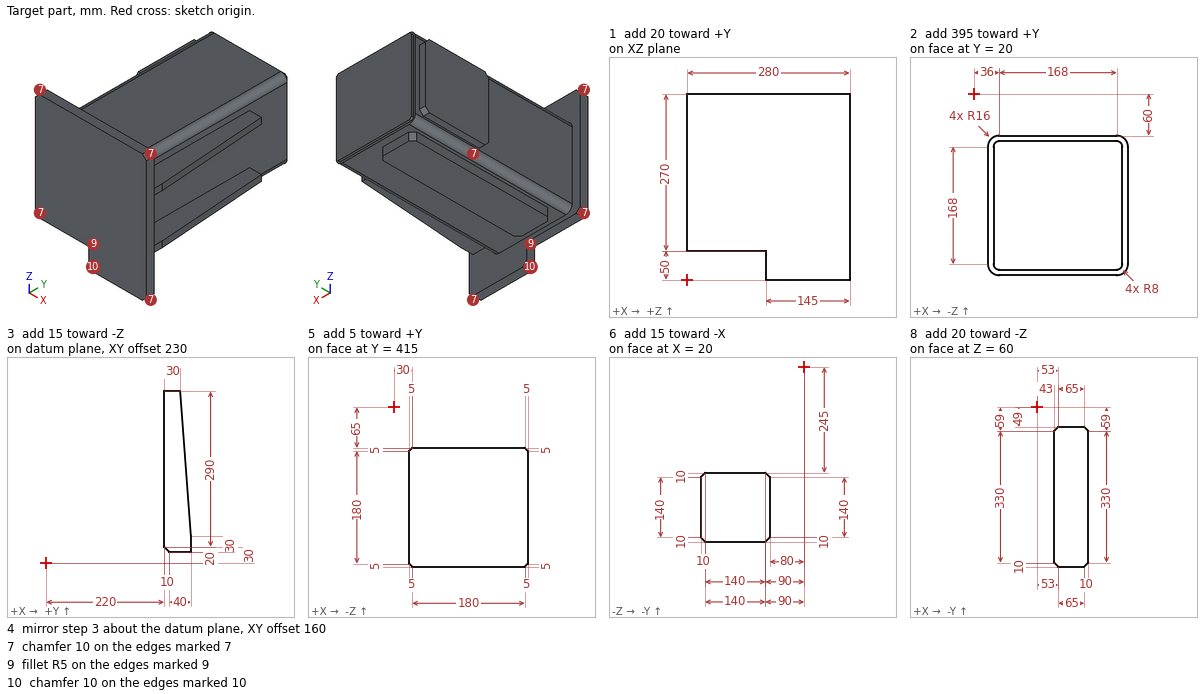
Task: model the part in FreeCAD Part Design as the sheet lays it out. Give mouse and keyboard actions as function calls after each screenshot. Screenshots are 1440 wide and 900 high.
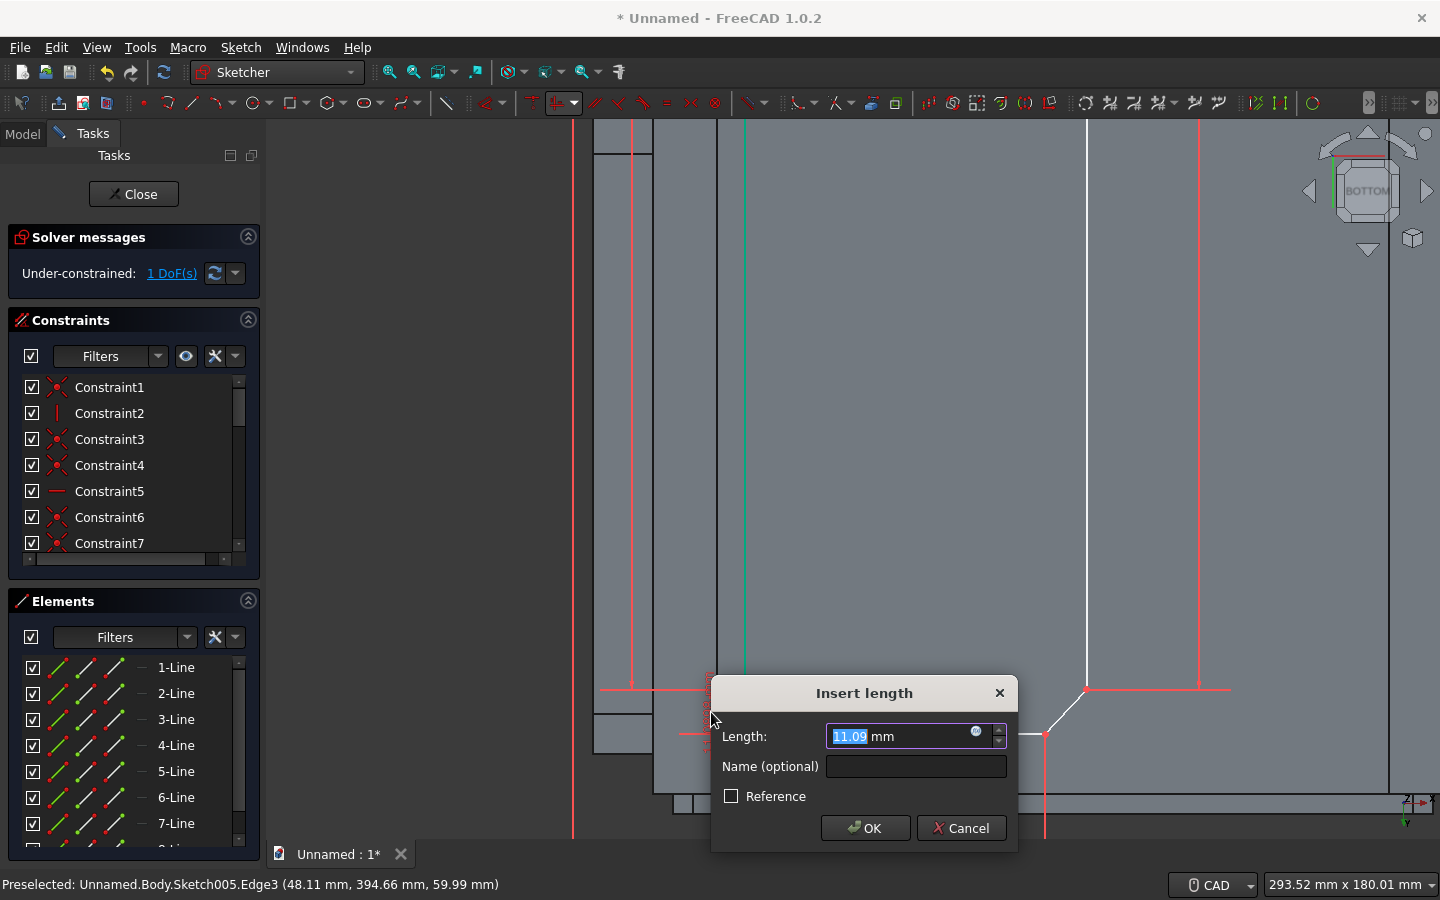
text(10)
key(Return)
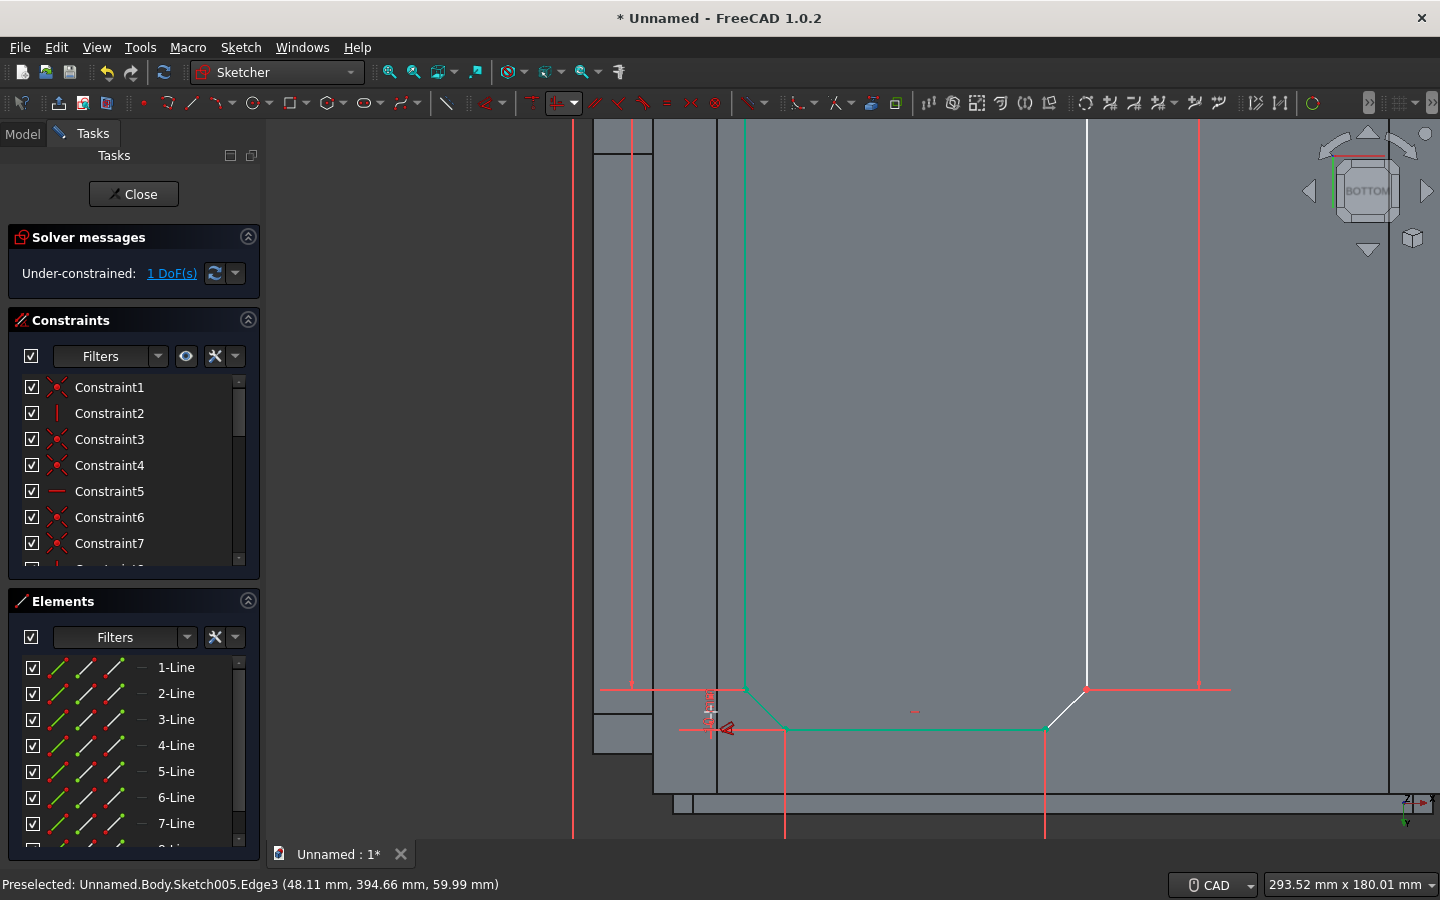
click(1057, 718)
click(1066, 764)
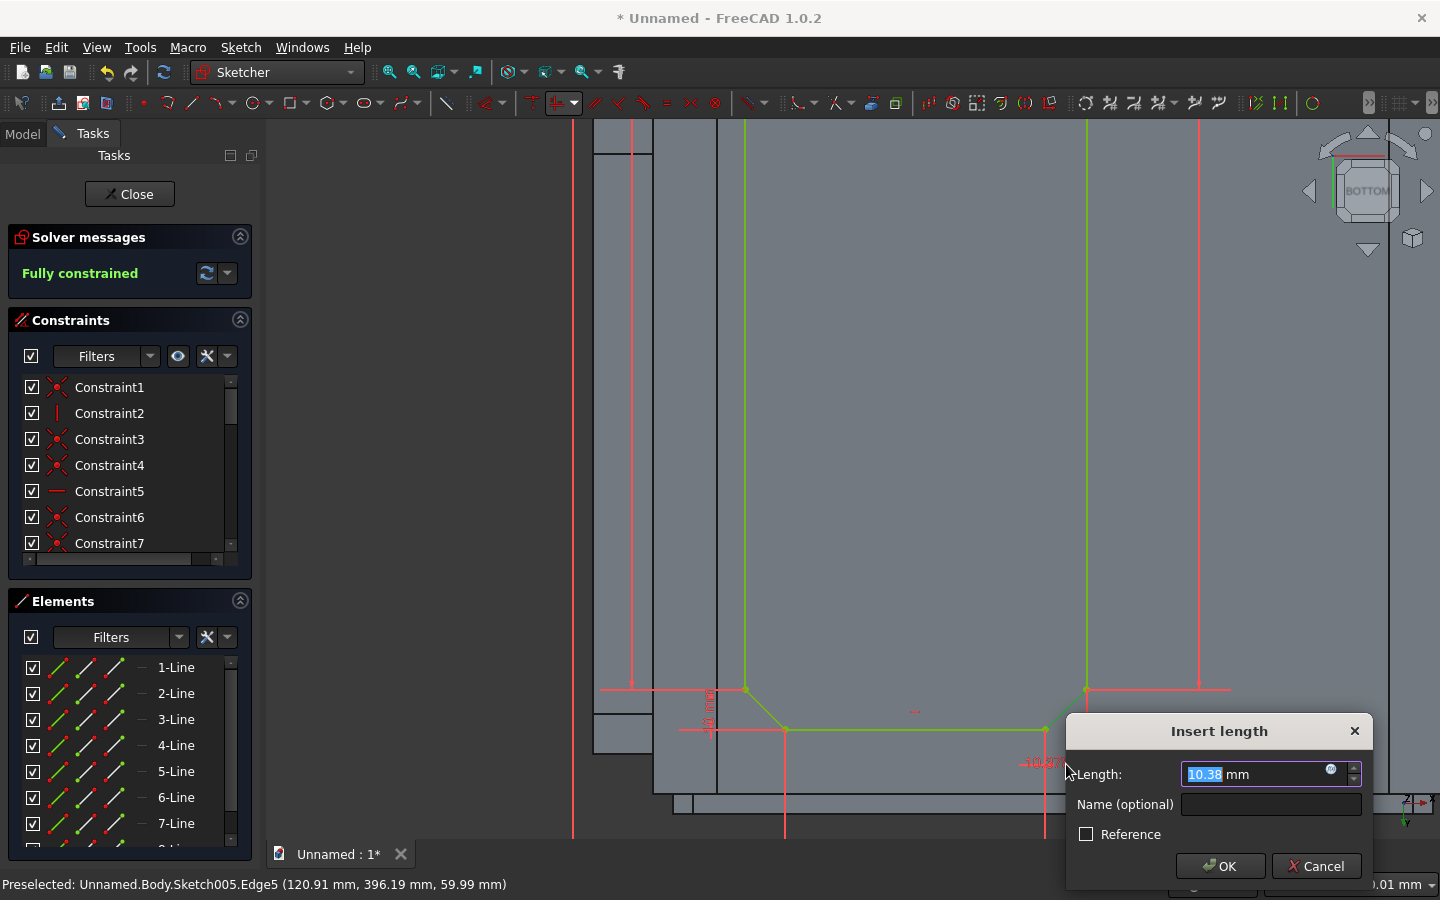
text(10)
key(Return)
key(Escape)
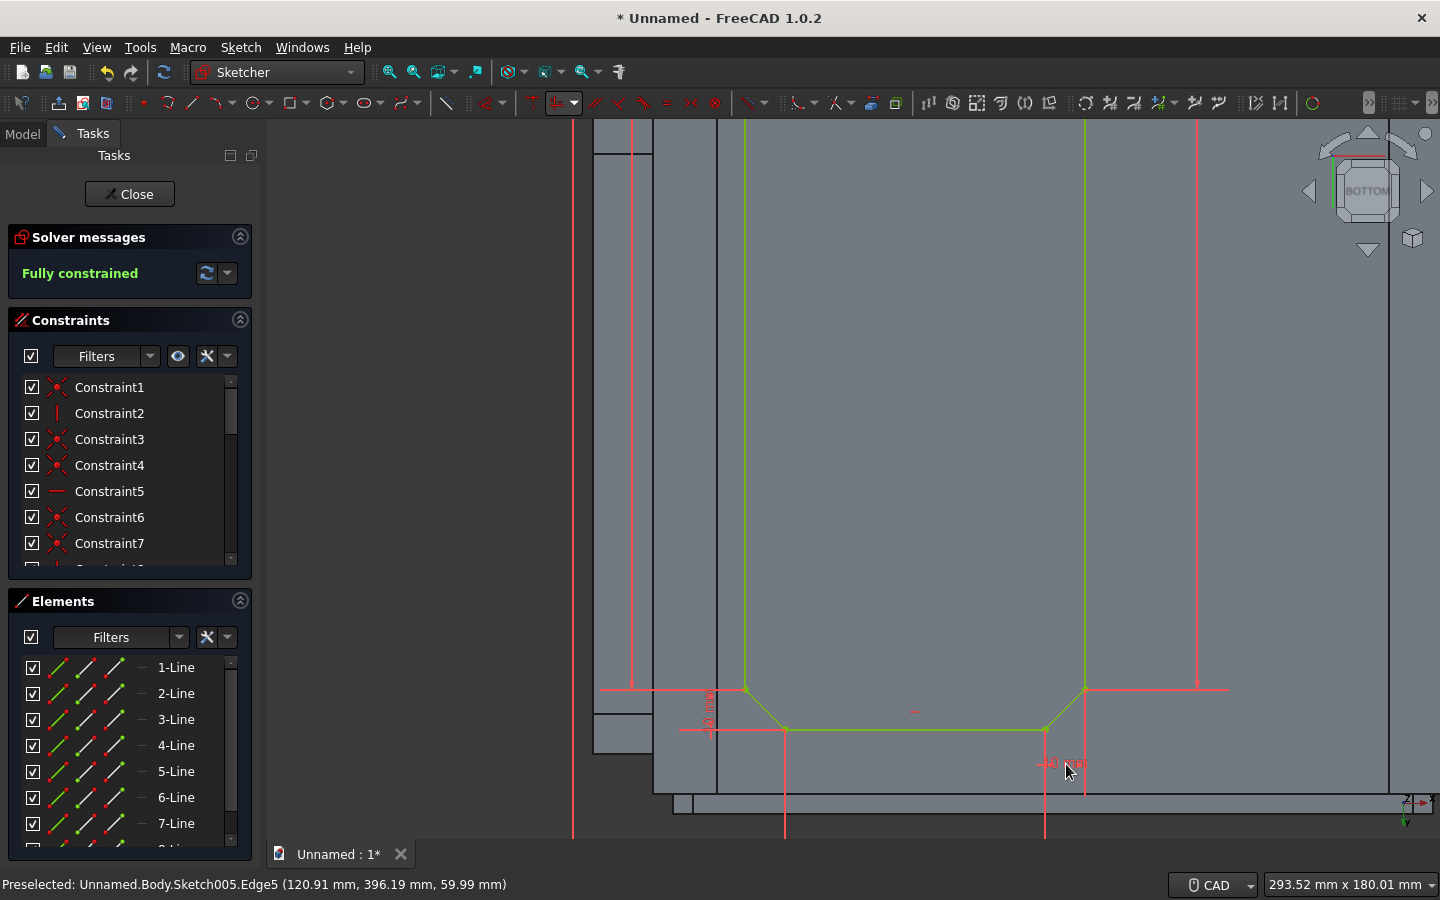
click(130, 194)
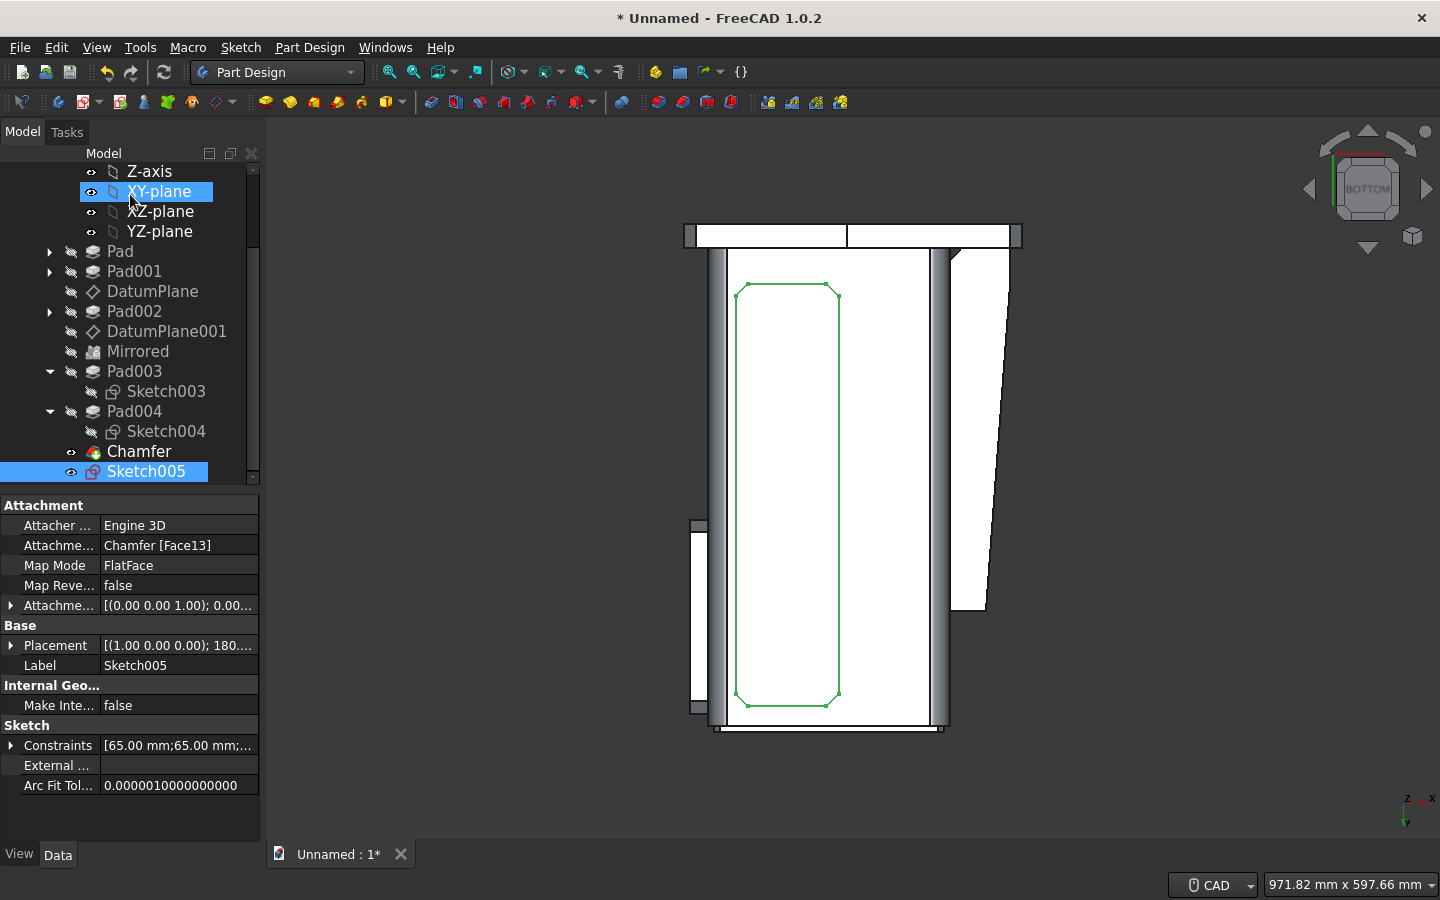
click(266, 102)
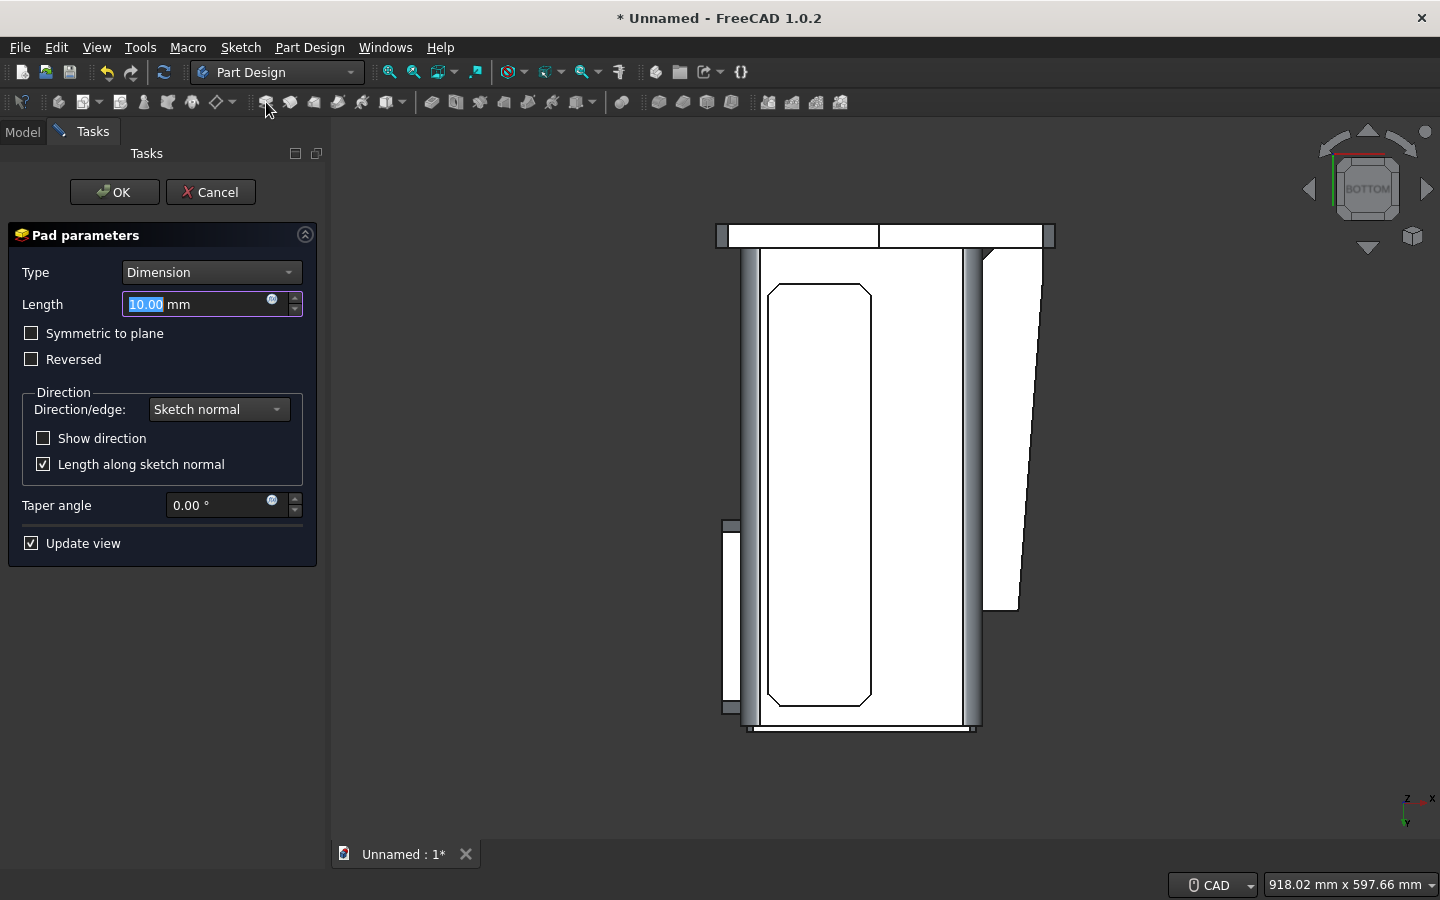
text(20)
key(Tab)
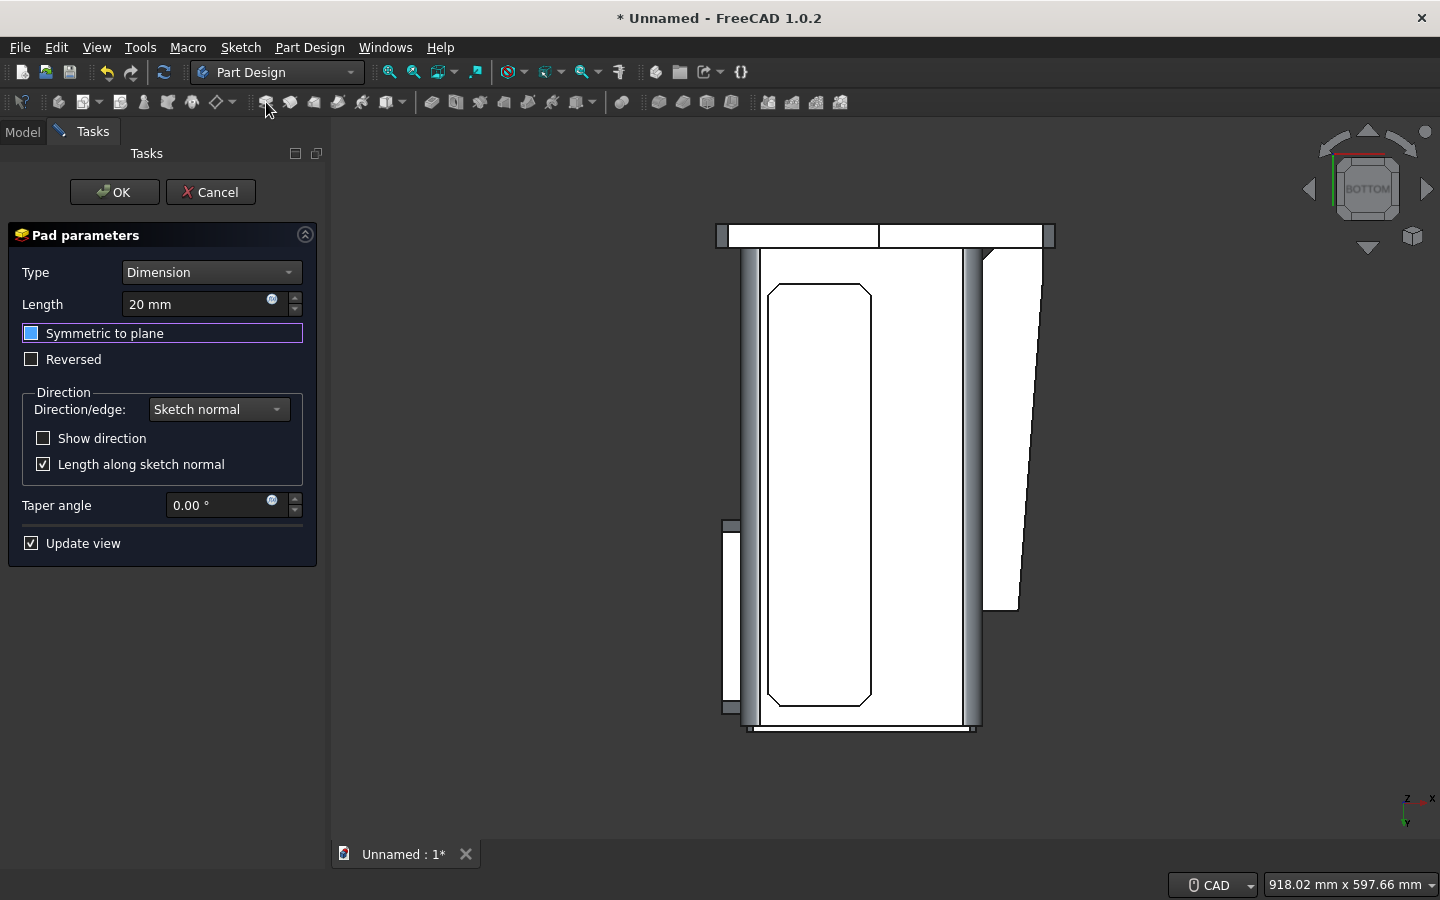
click(115, 192)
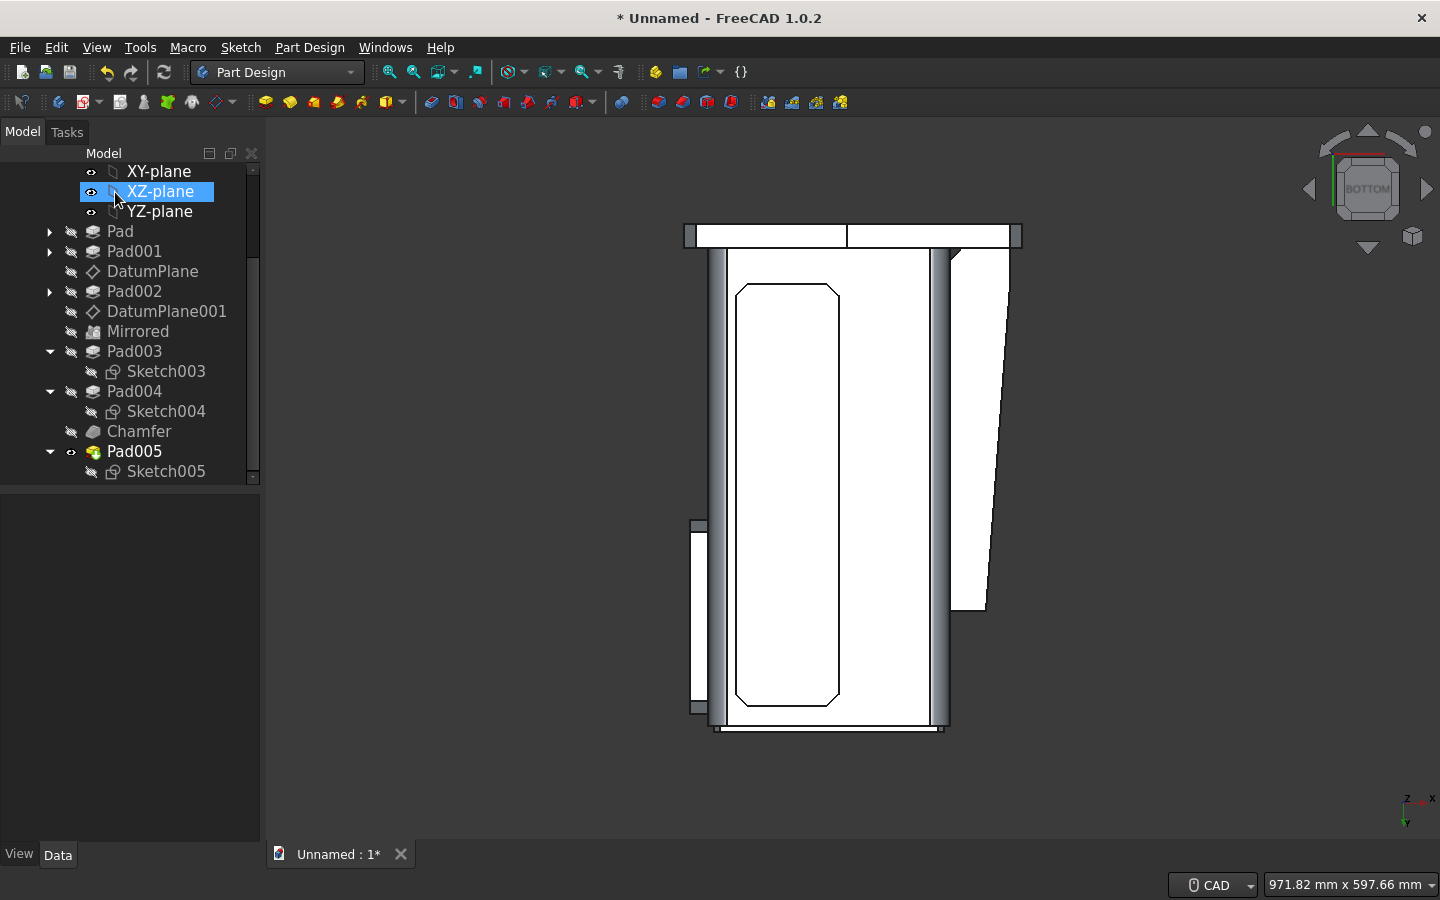
key(0)